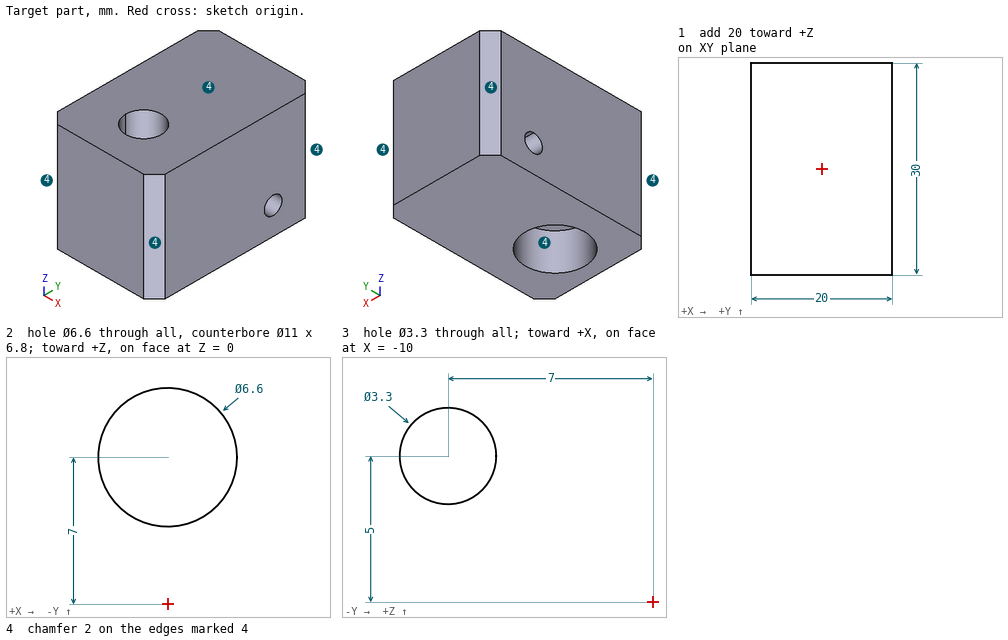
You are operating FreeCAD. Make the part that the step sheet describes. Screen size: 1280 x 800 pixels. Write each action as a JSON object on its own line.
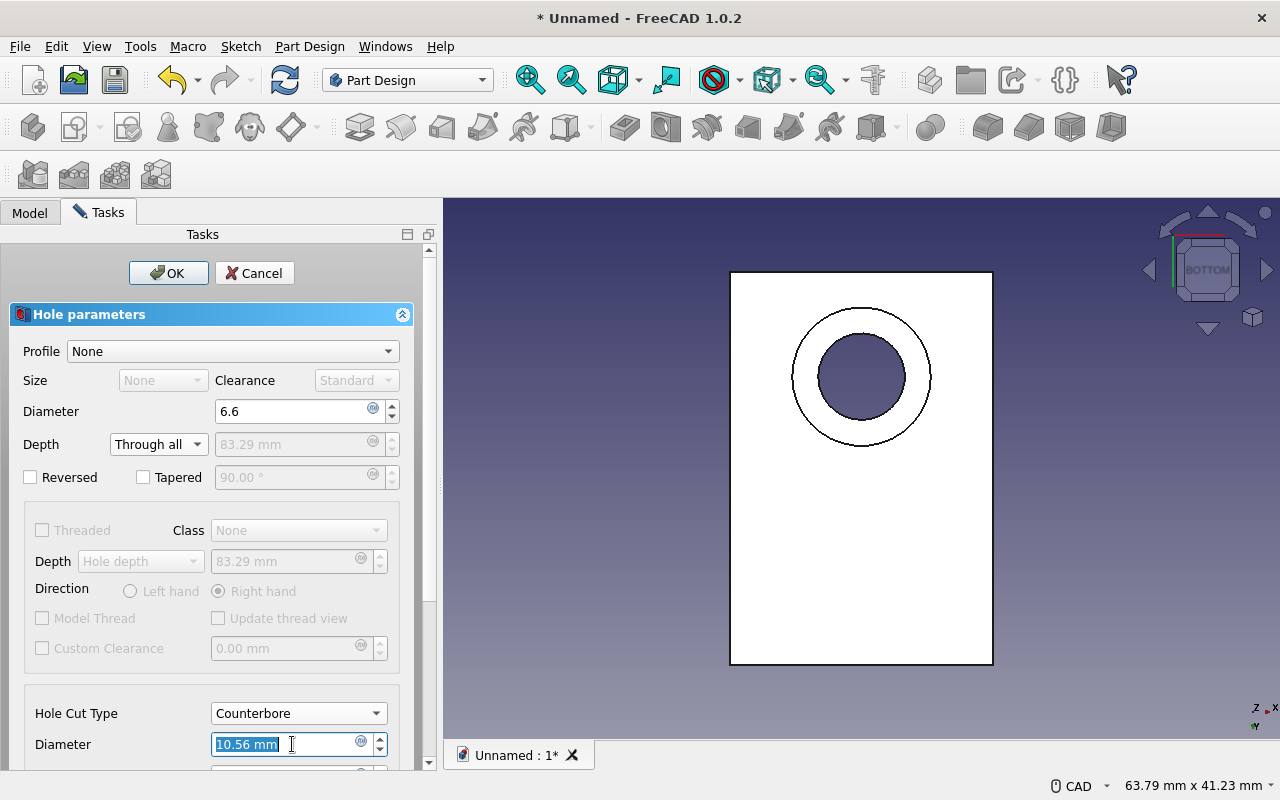
{"action": "type", "text": "11"}
{"action": "key", "text": "Tab"}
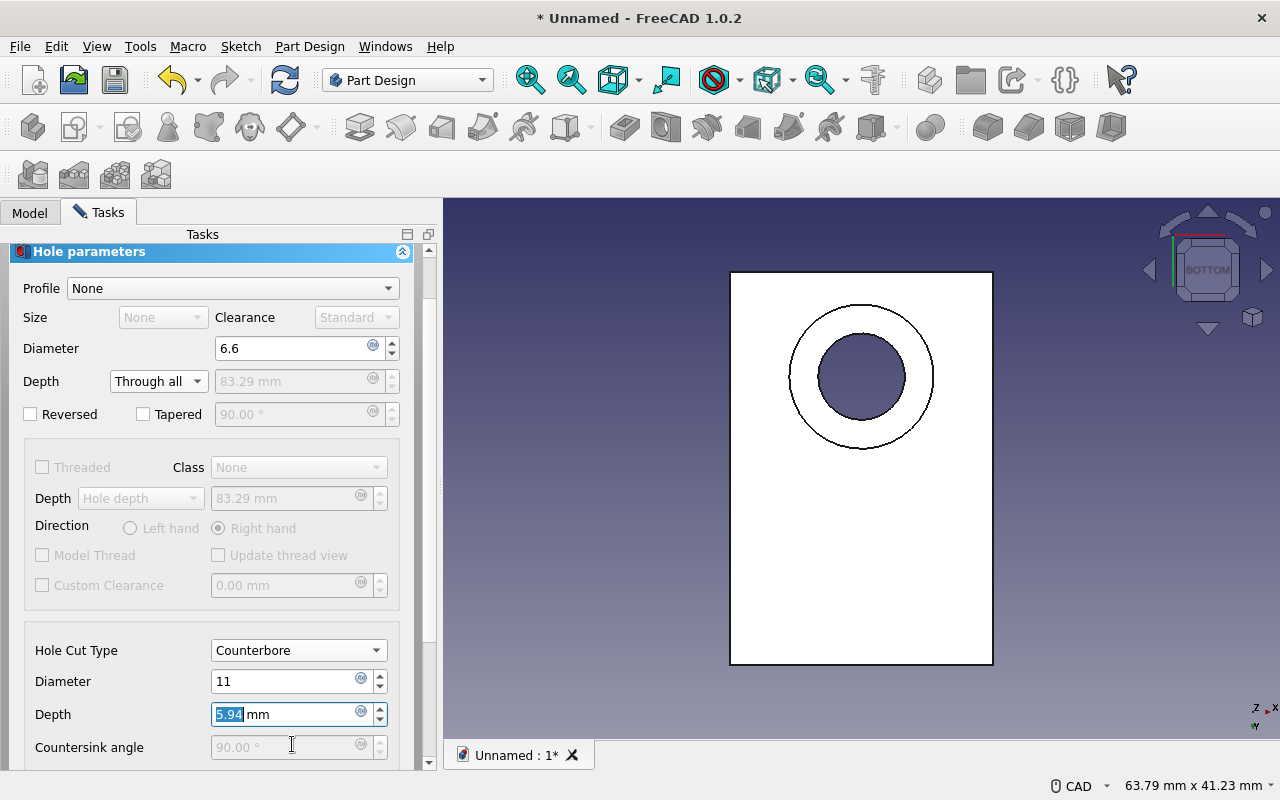
{"action": "type", "text": "6.8"}
{"action": "key", "text": "Tab"}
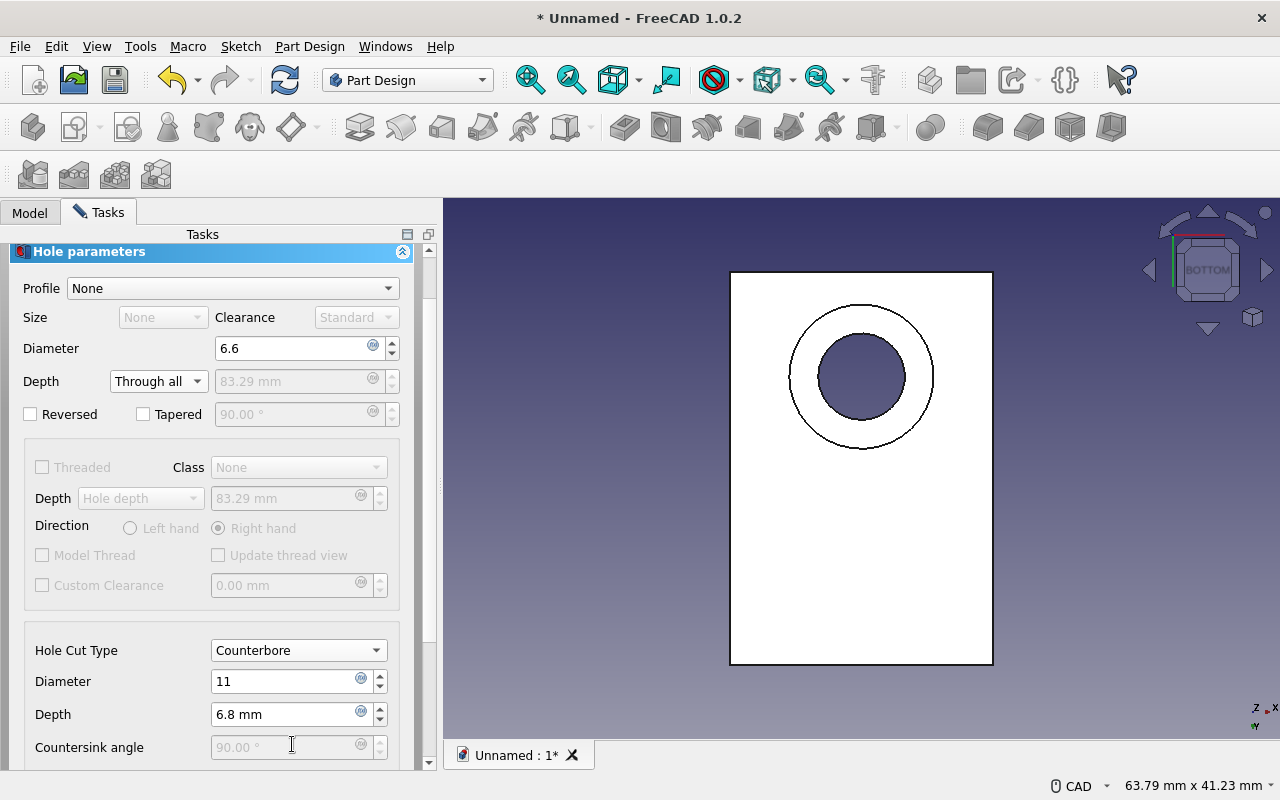
{"action": "scroll", "coordinate": [429, 507], "scroll_direction": "up", "scroll_amount": 2}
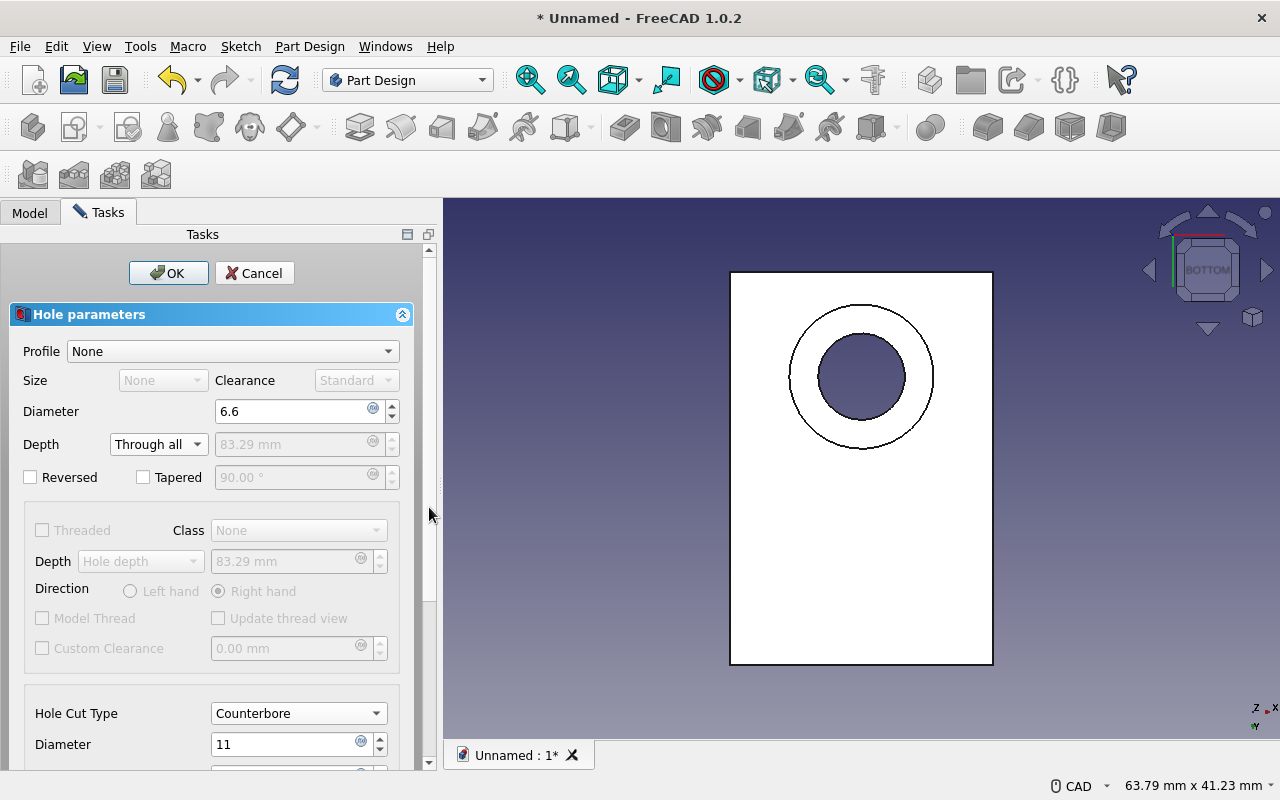
{"action": "left_click", "coordinate": [169, 273]}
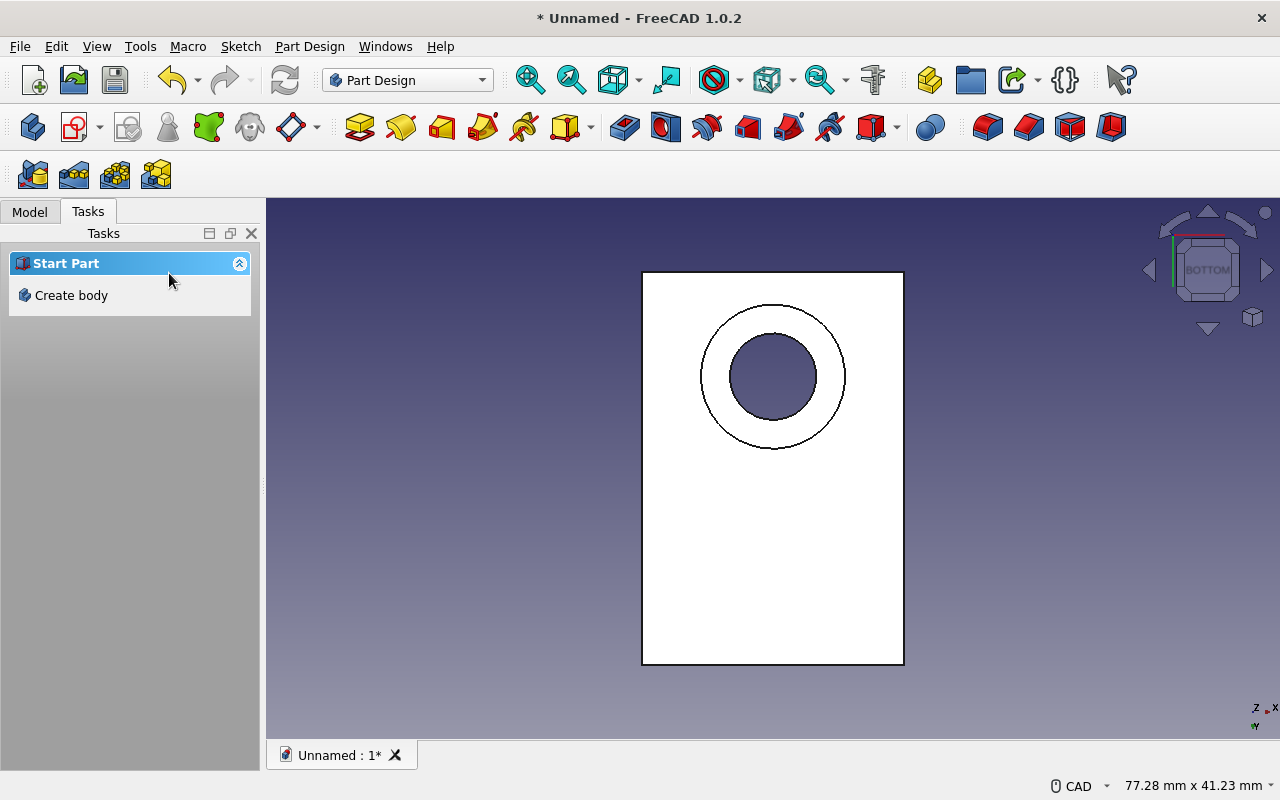
{"action": "key", "text": "6"}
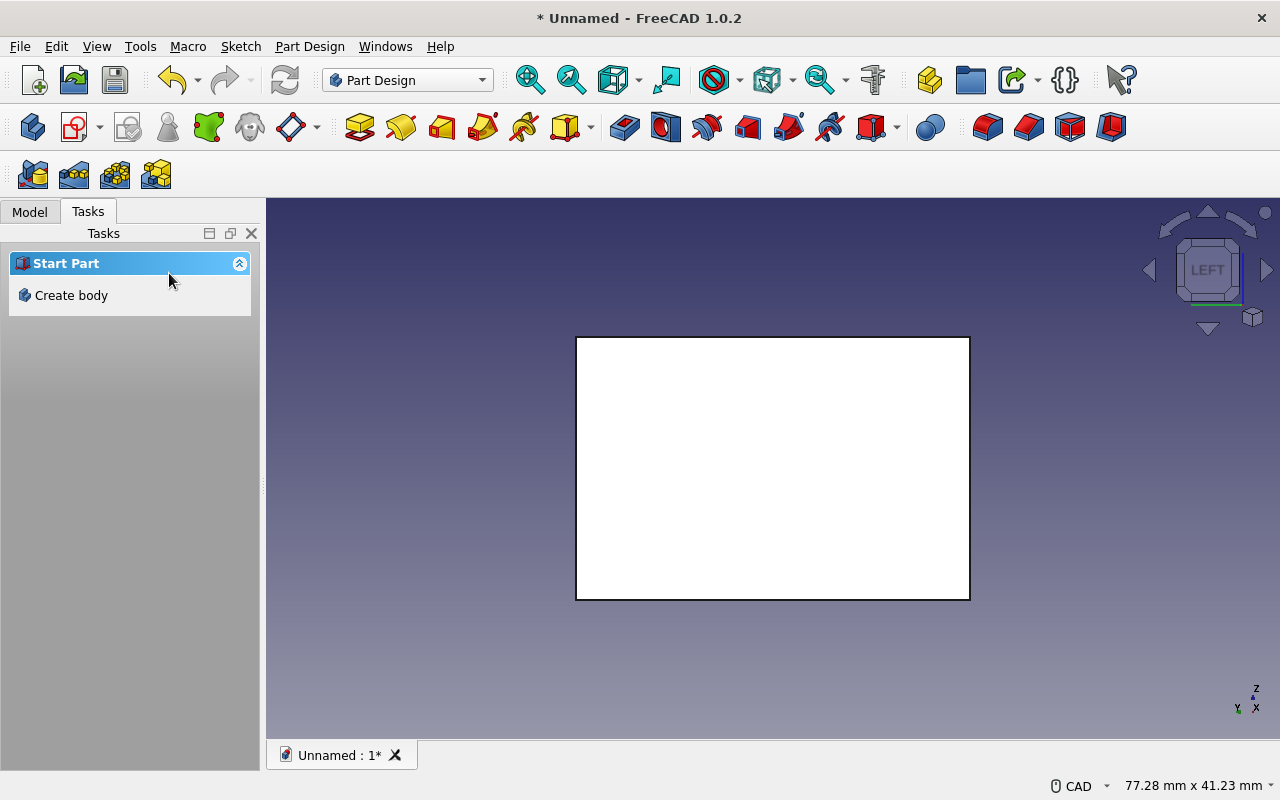
{"action": "left_click", "coordinate": [717, 467]}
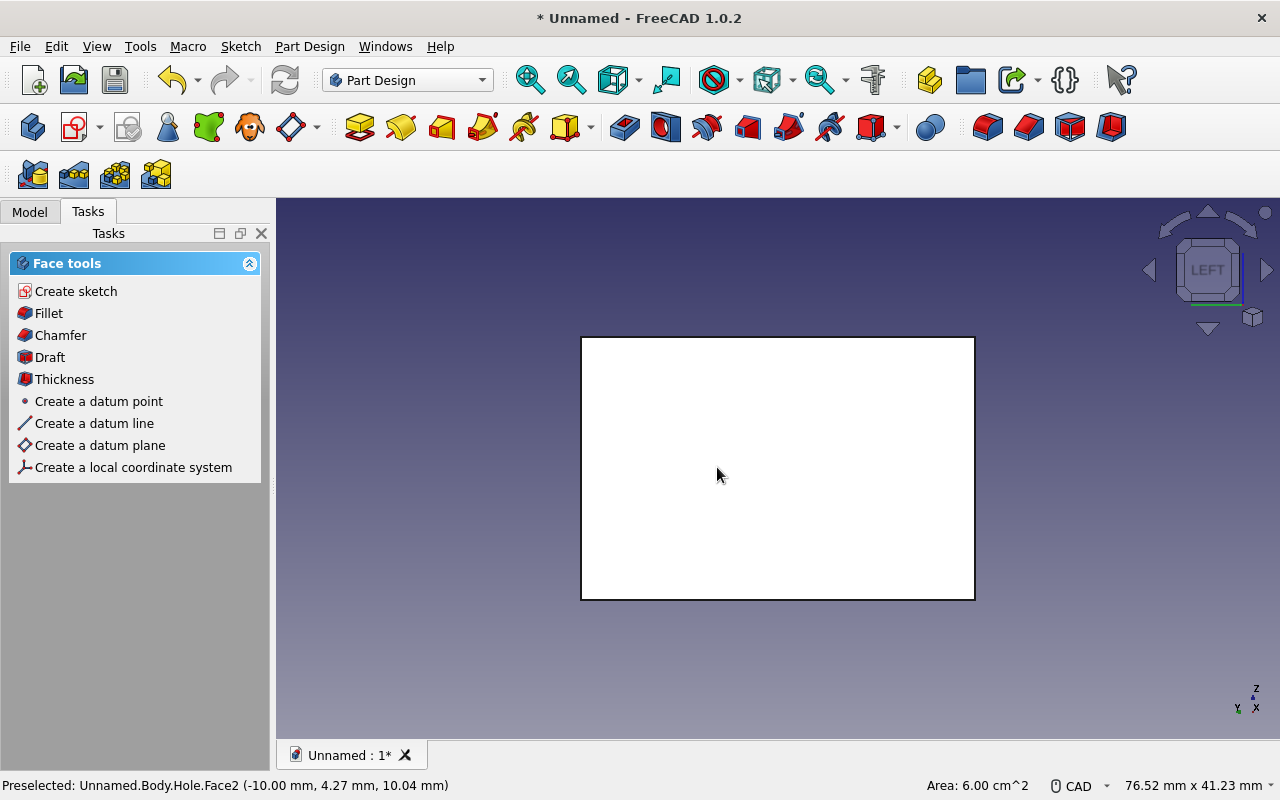
{"action": "left_click", "coordinate": [74, 128]}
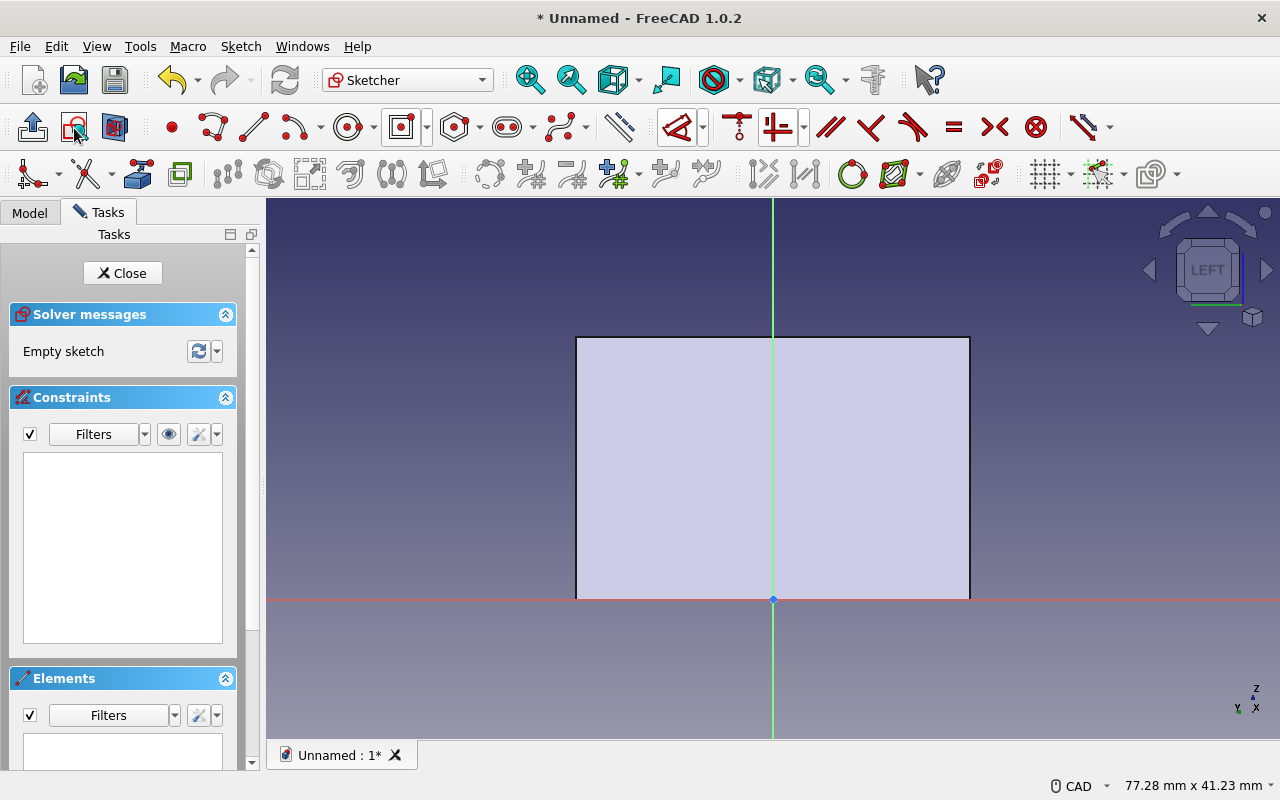
{"action": "scroll", "coordinate": [677, 544], "scroll_direction": "up", "scroll_amount": 10}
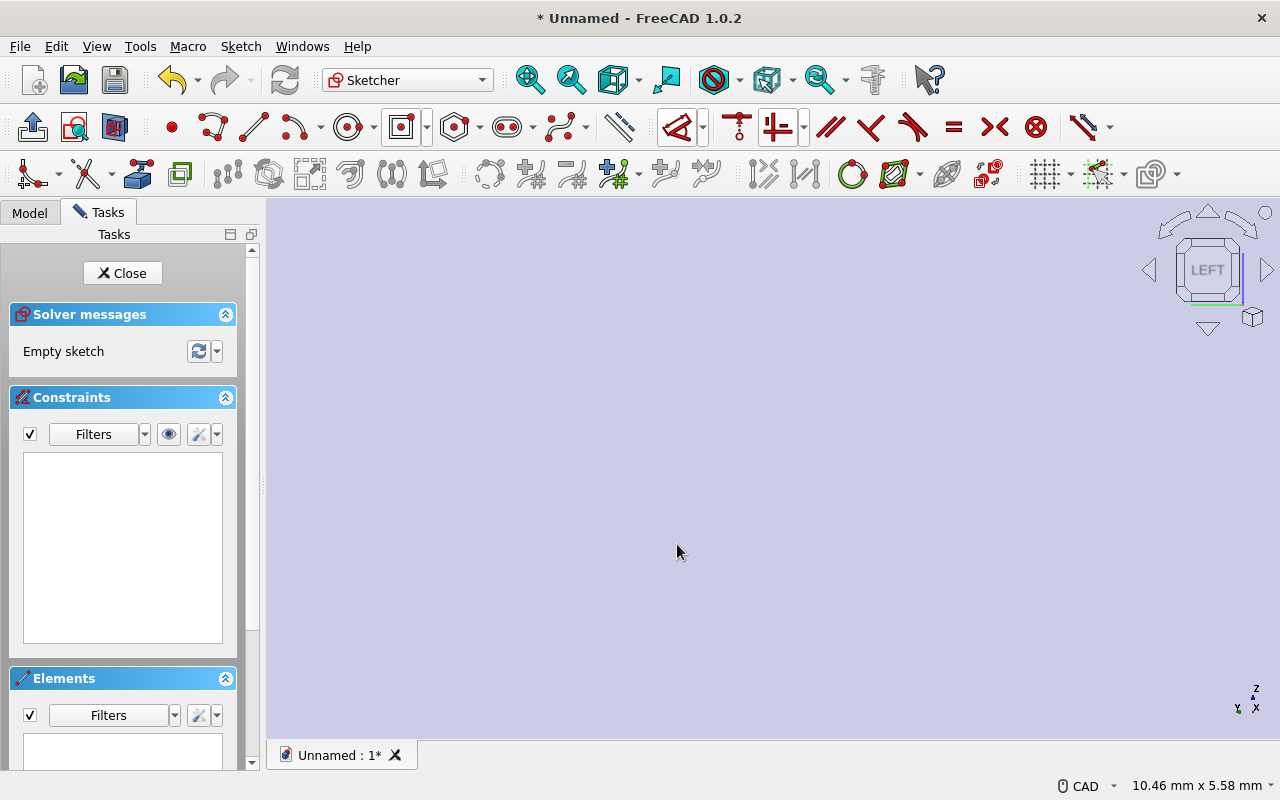
{"action": "key", "text": "g c"}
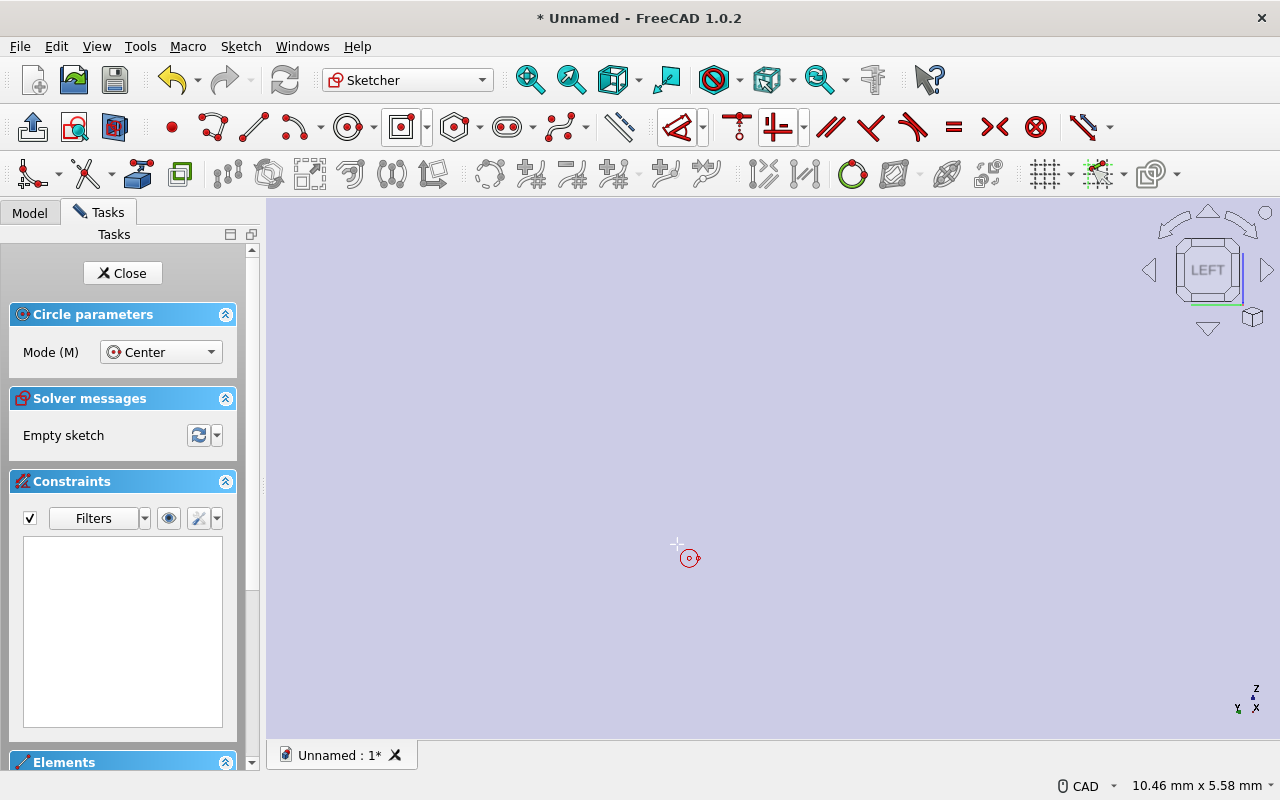
{"action": "left_click", "coordinate": [705, 467]}
{"action": "left_click", "coordinate": [818, 354]}
{"action": "key", "text": "Escape"}